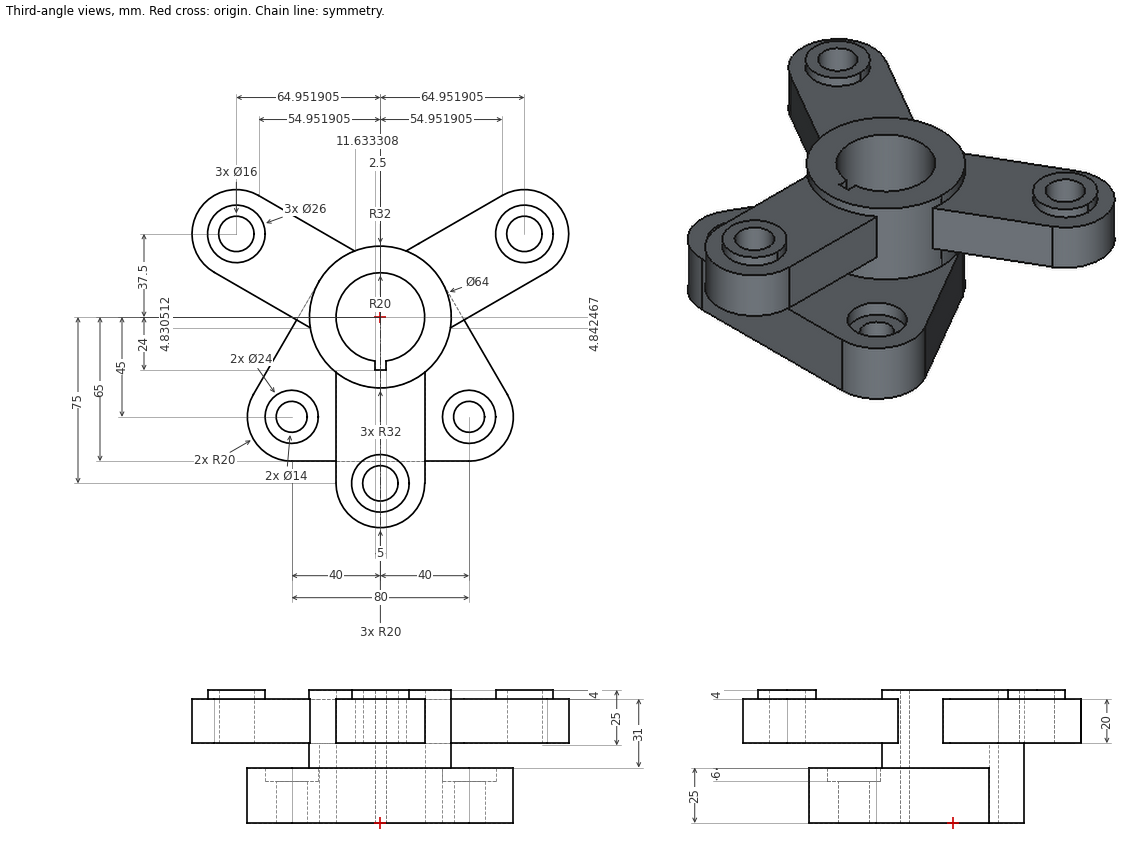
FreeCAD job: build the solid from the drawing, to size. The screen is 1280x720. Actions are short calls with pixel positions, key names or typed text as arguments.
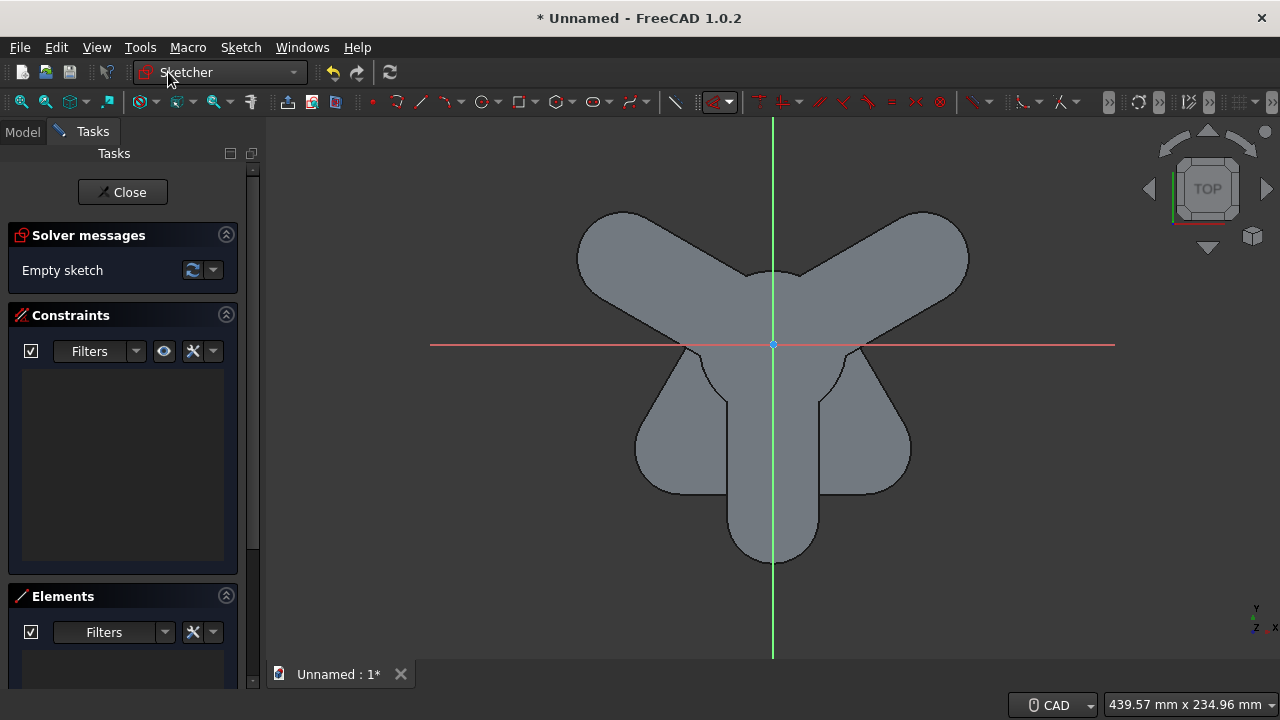
scroll(829, 309, up, 4)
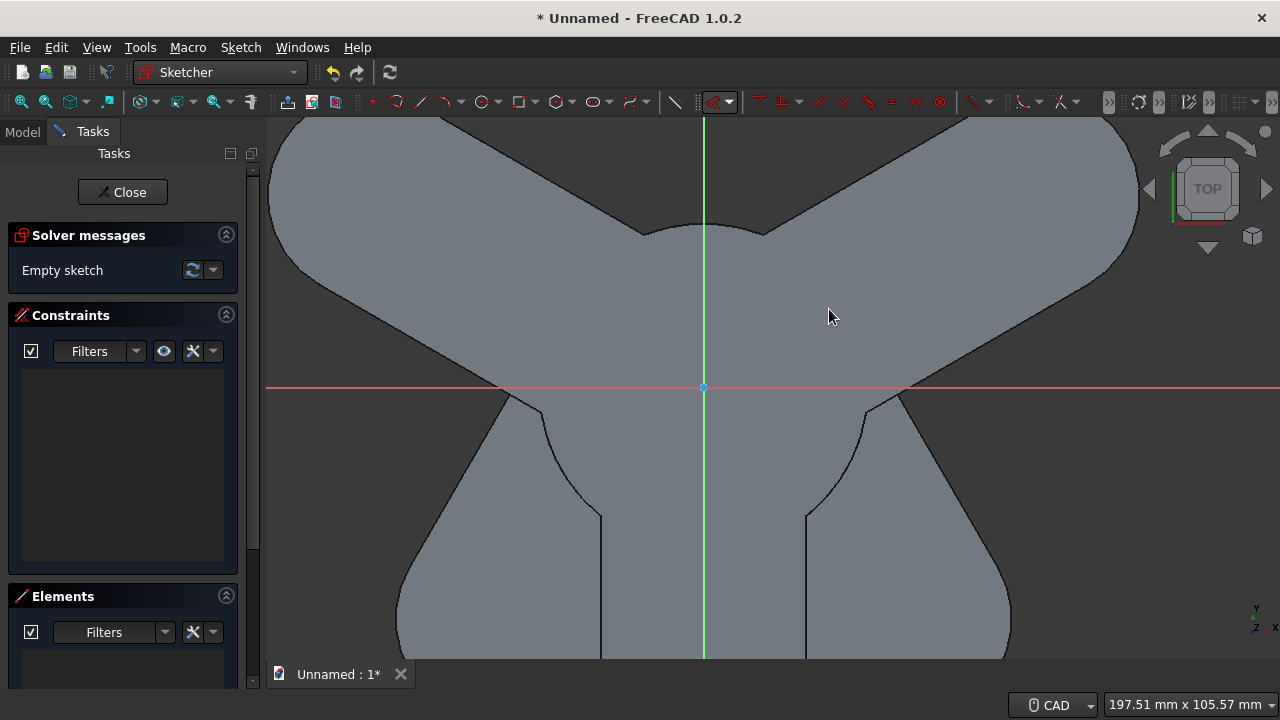
click(482, 102)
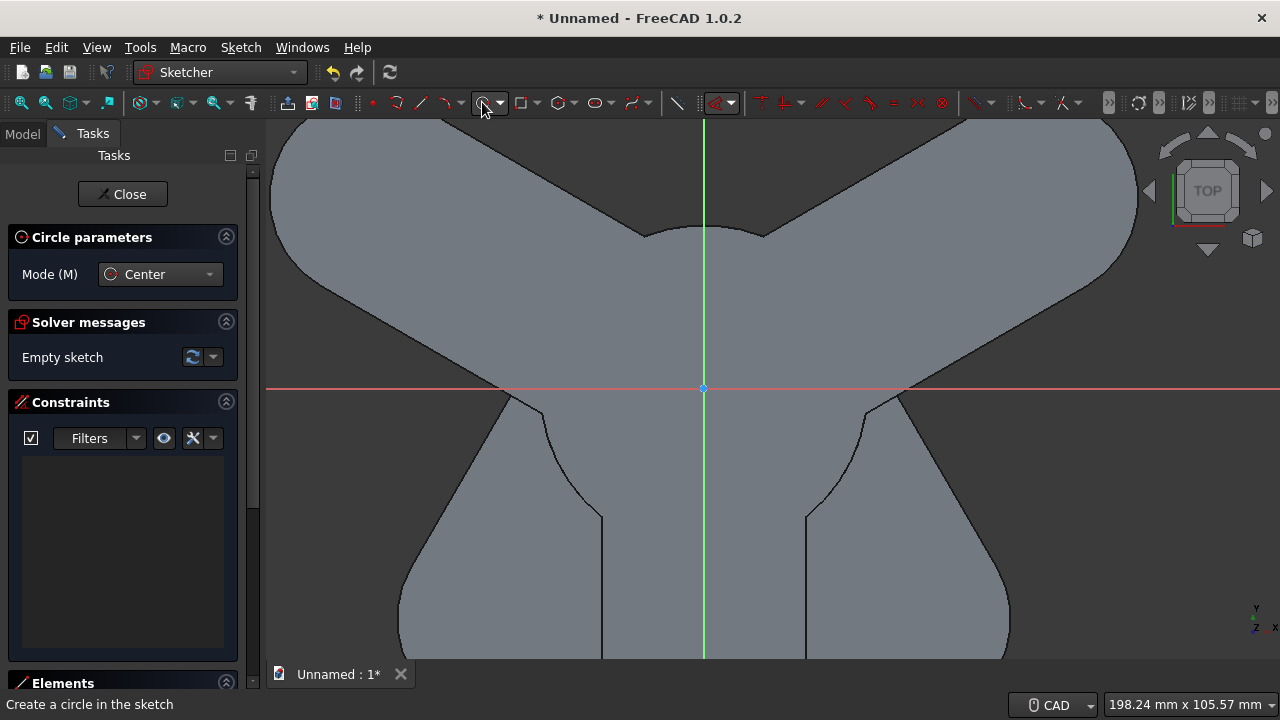
click(704, 389)
click(820, 273)
key(Escape)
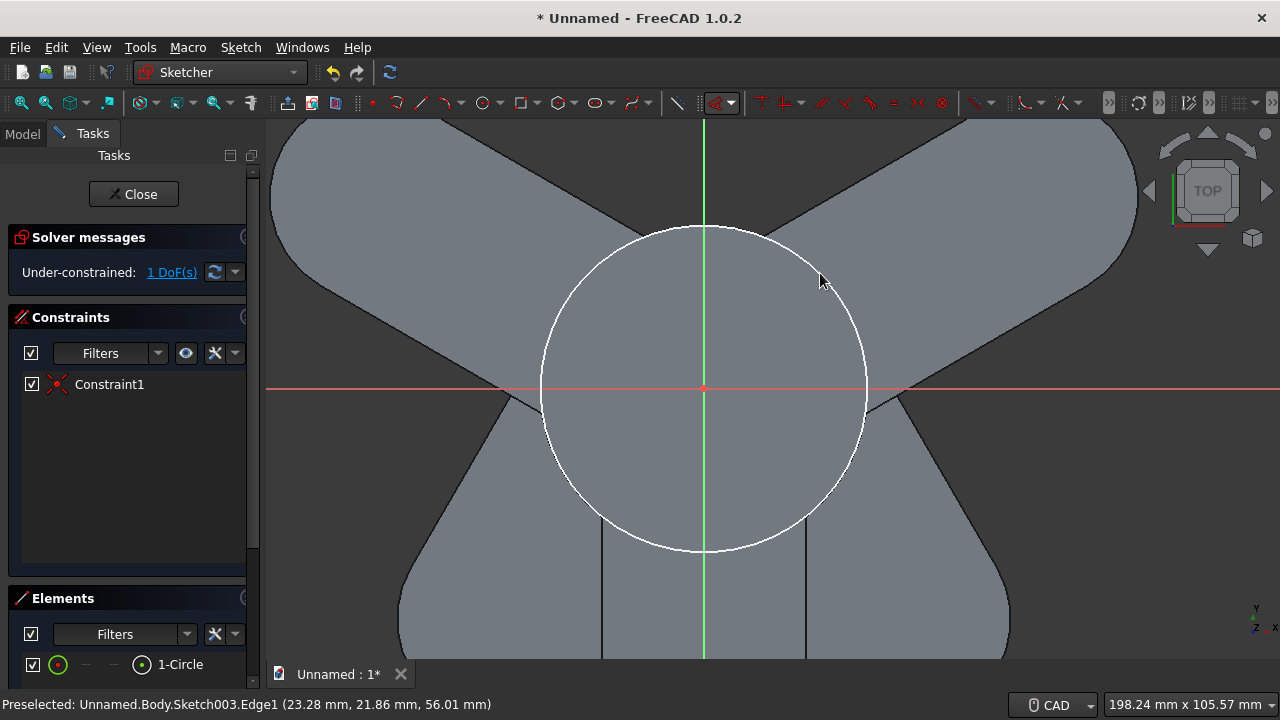
click(819, 273)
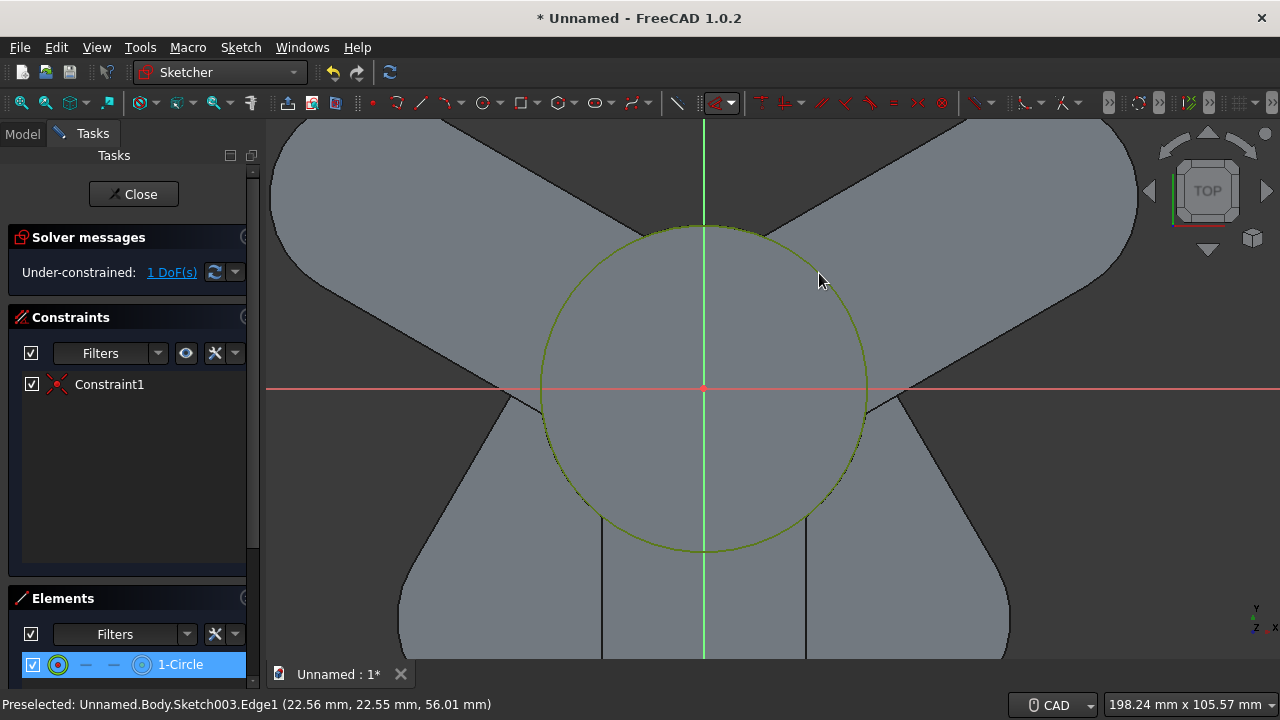
key(k)
key(o)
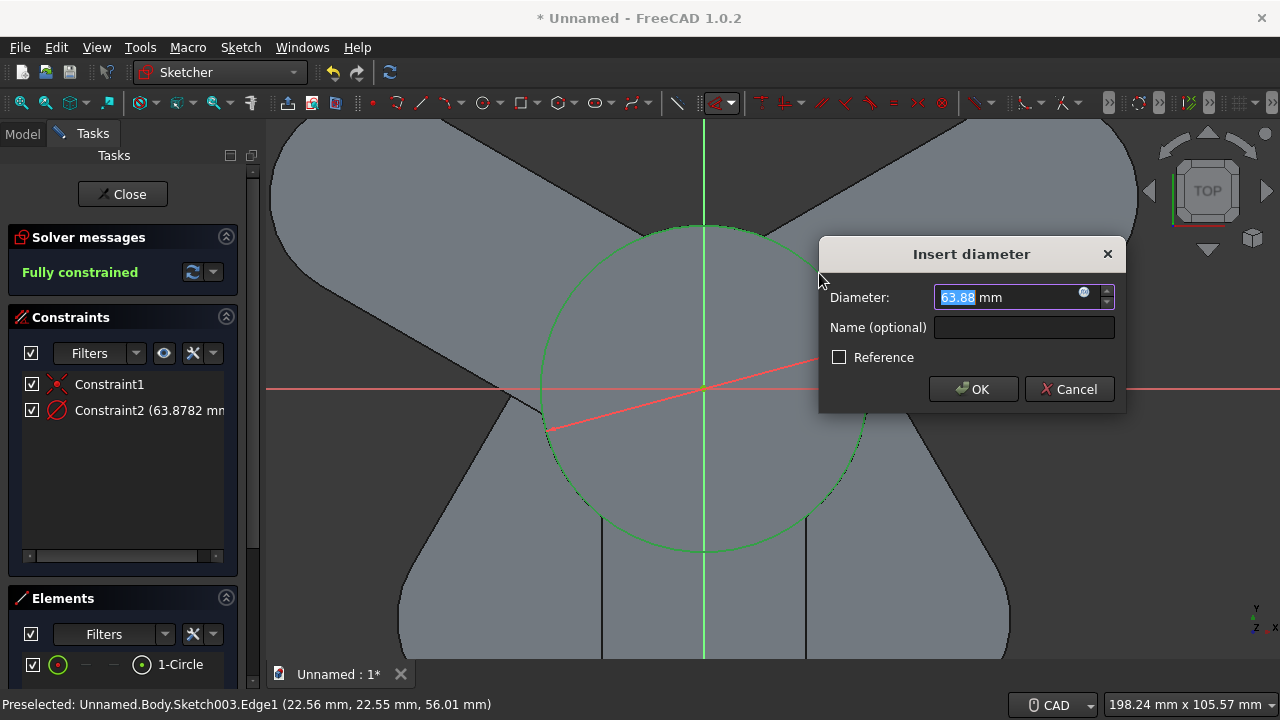
text(64)
key(Return)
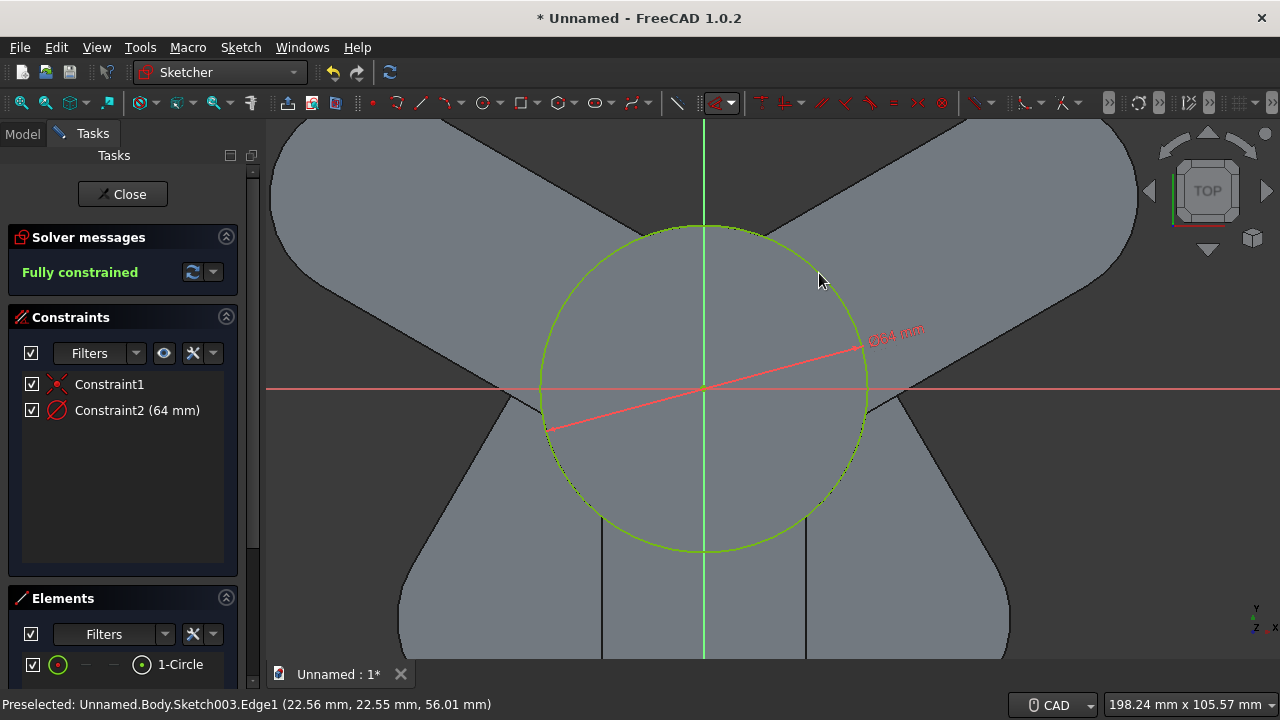
click(123, 194)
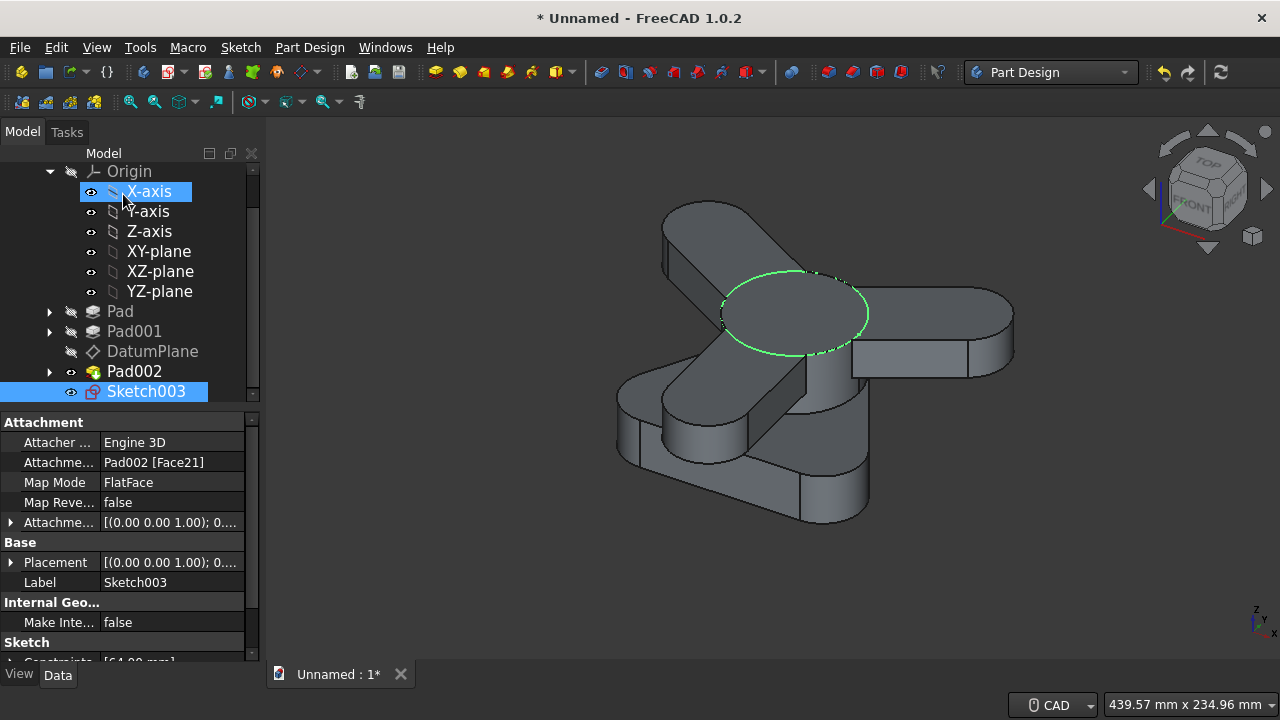
click(436, 72)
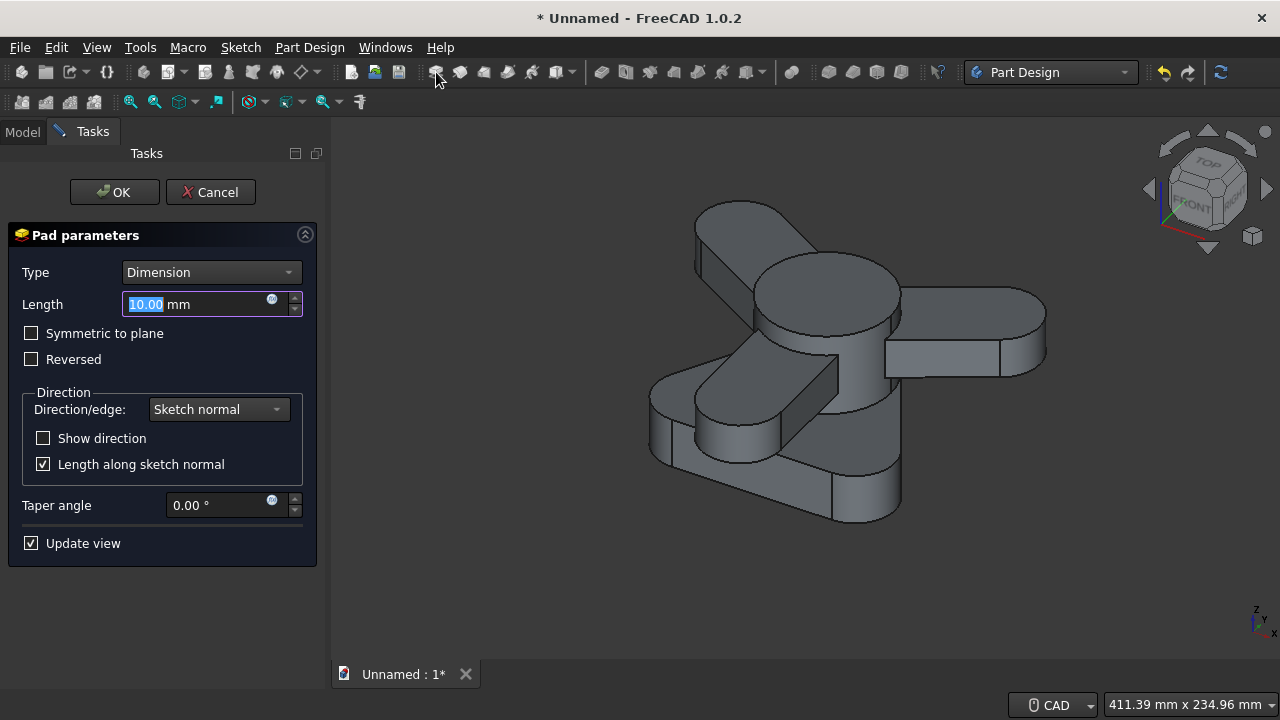
text(4)
key(Tab)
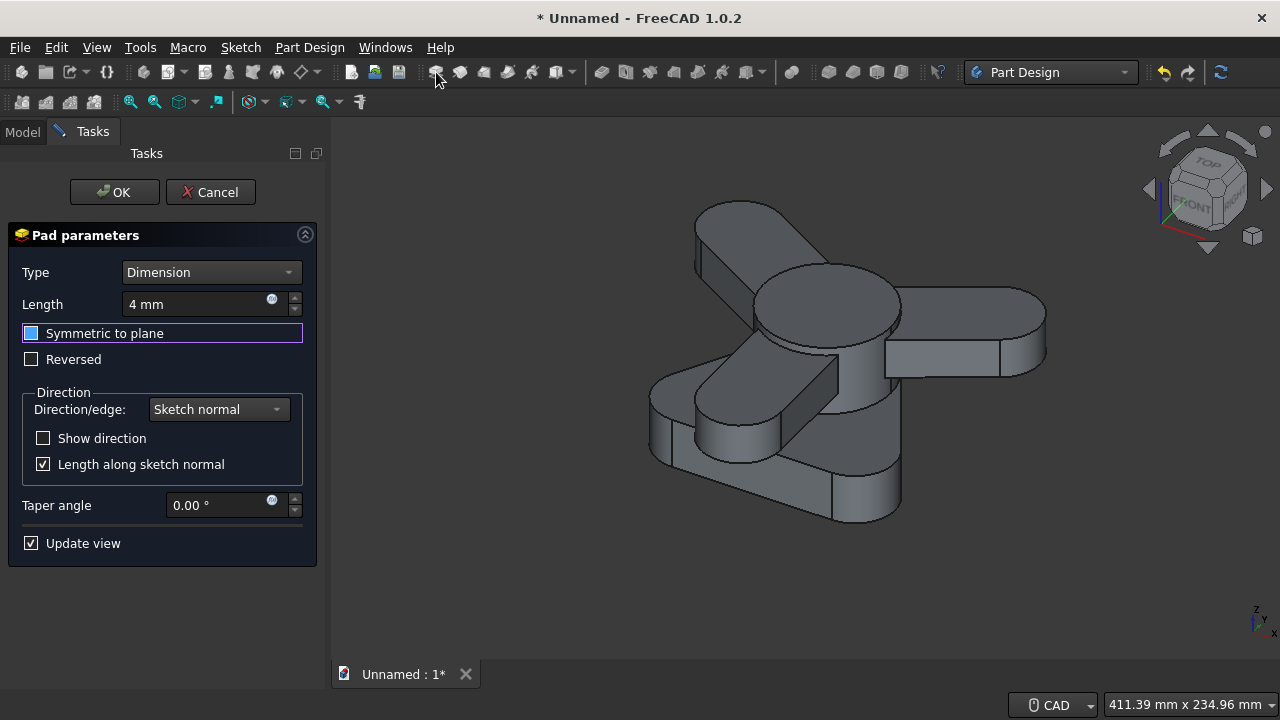
click(115, 192)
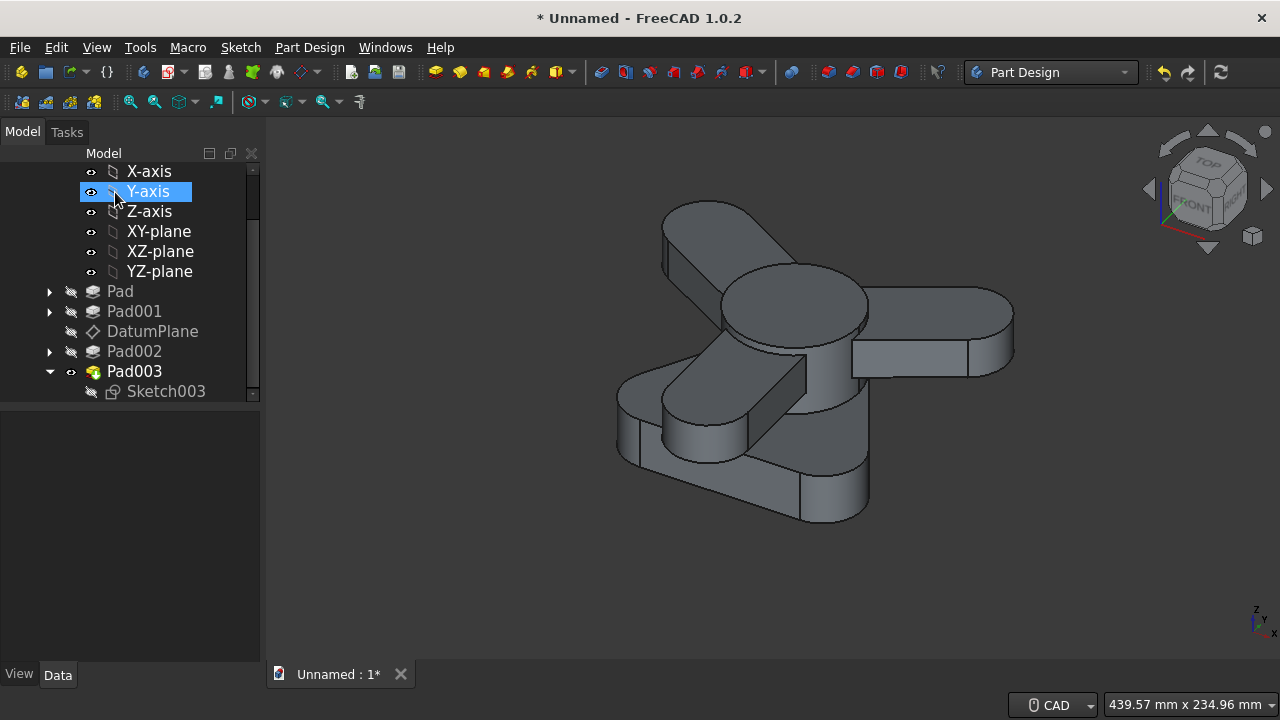
click(953, 311)